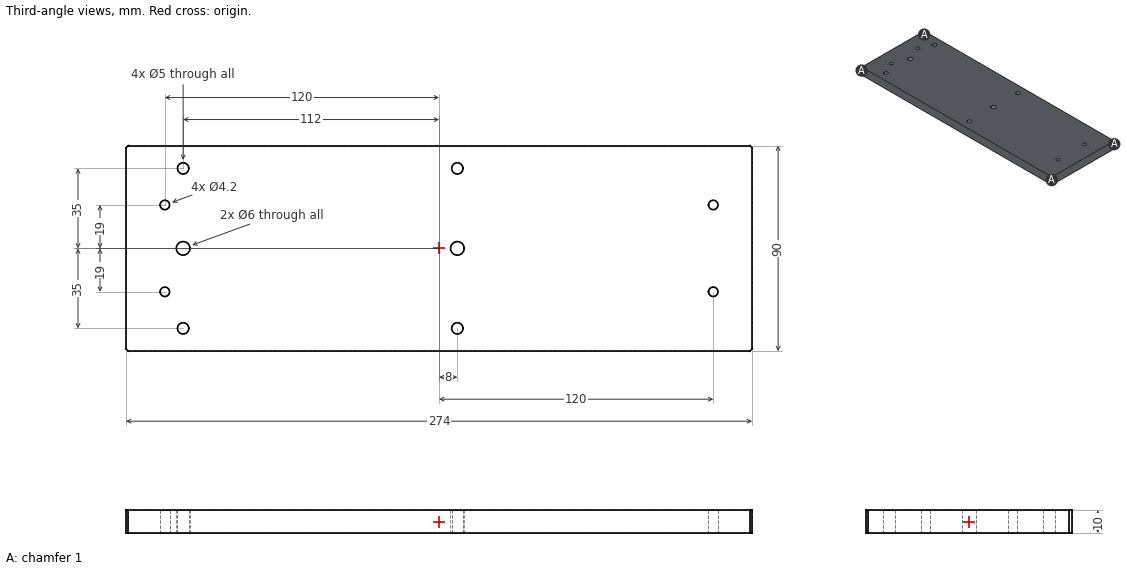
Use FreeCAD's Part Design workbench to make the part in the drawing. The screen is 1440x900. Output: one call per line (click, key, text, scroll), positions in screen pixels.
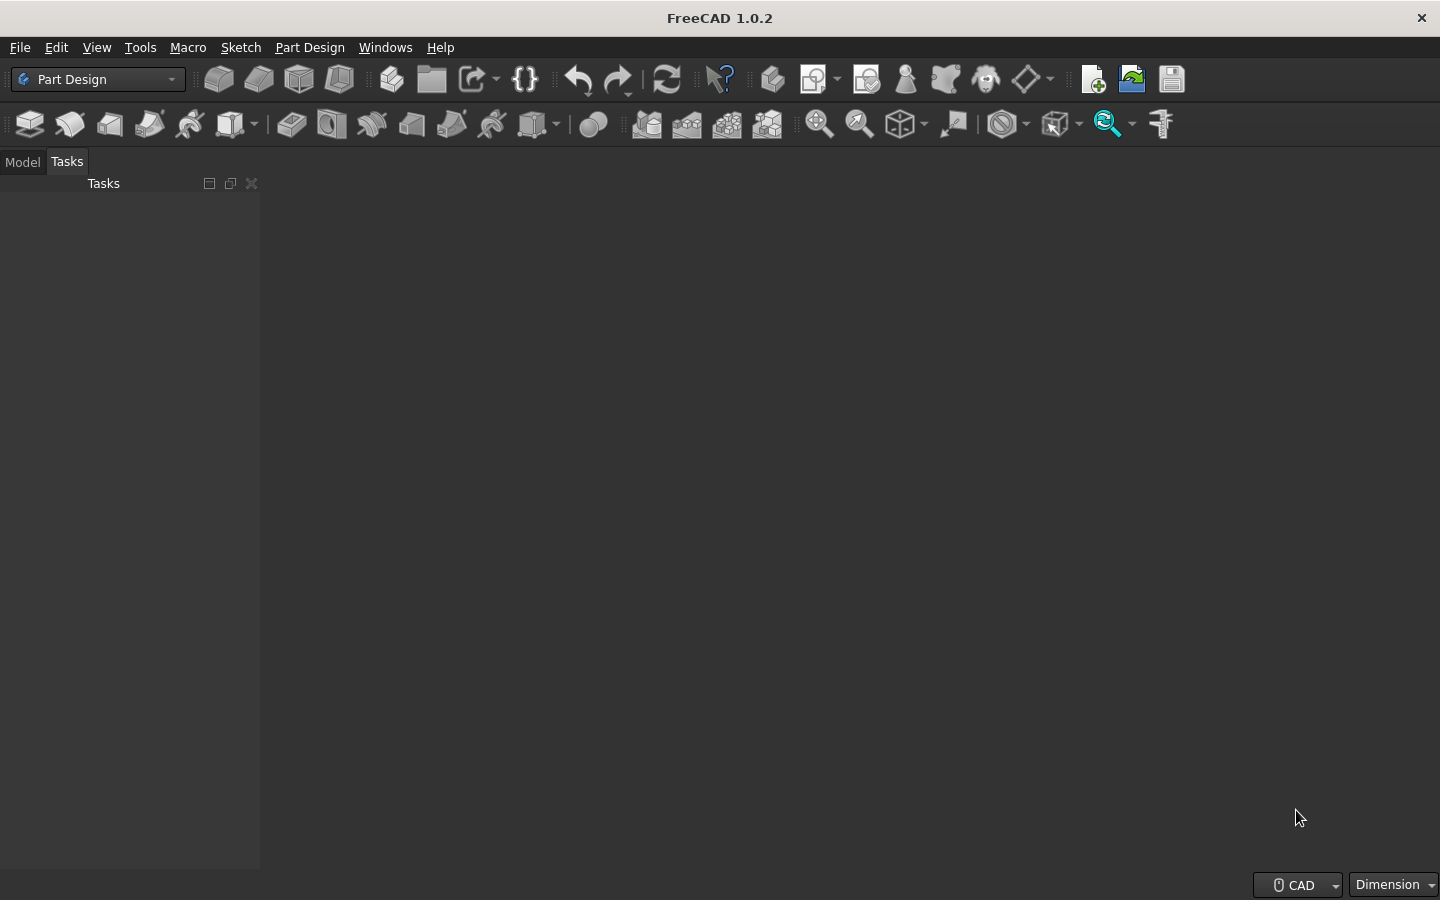
key(ctrl+n)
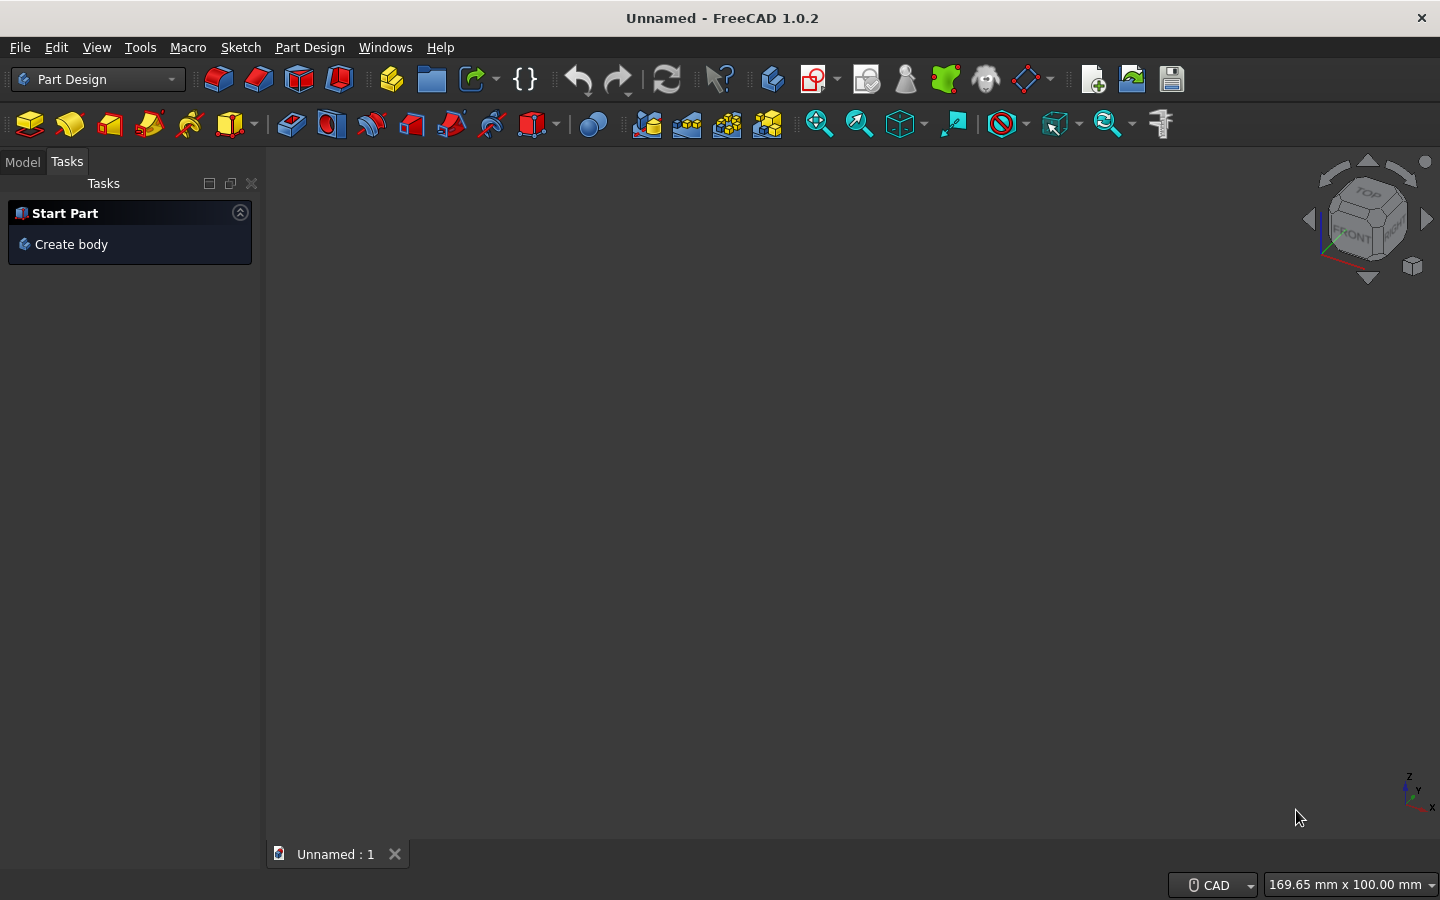
click(814, 80)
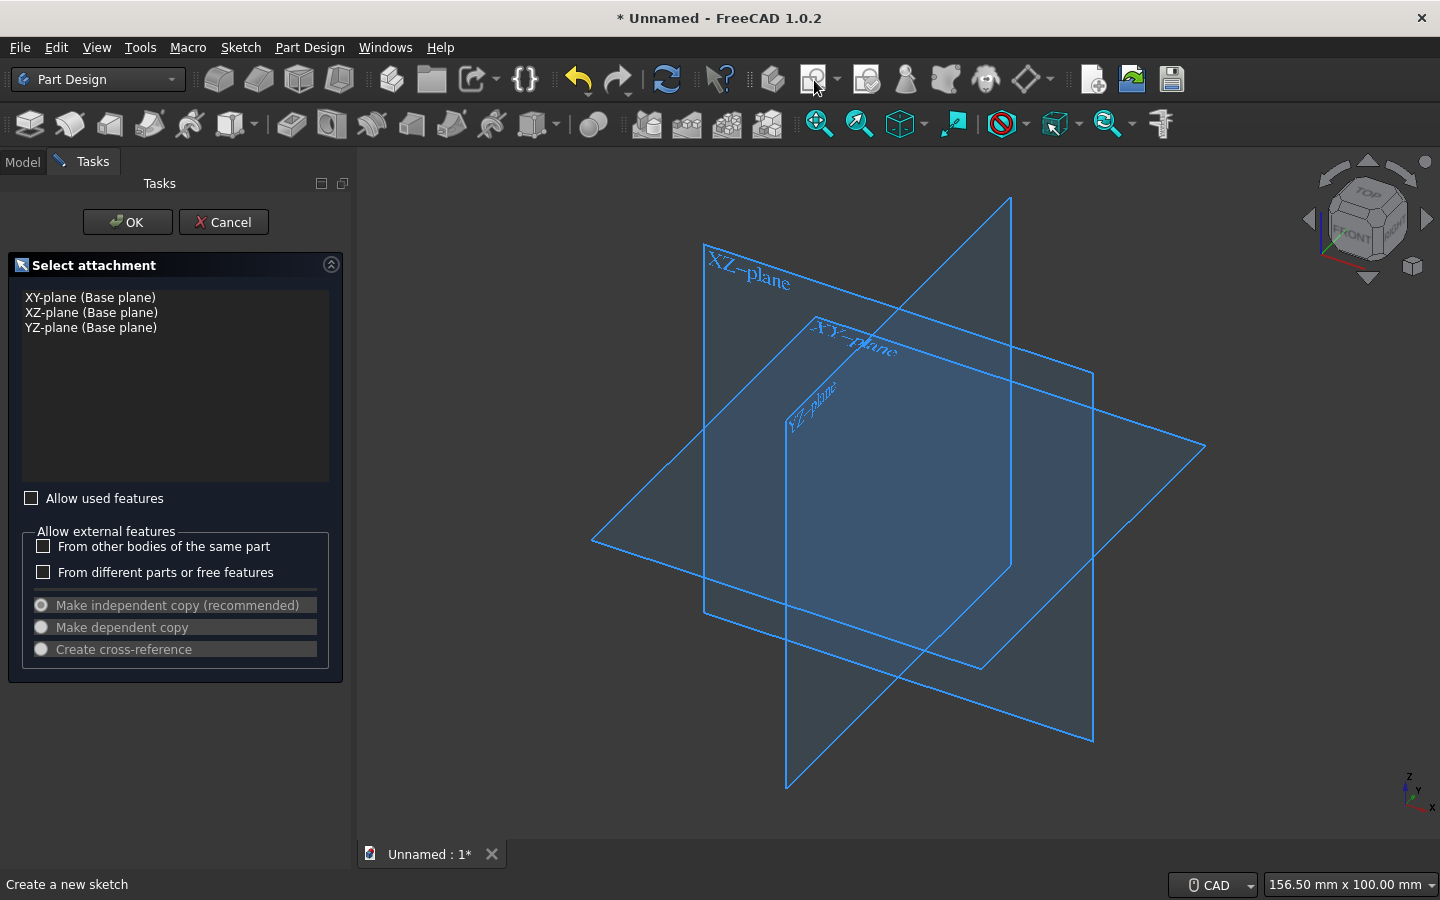
click(82, 298)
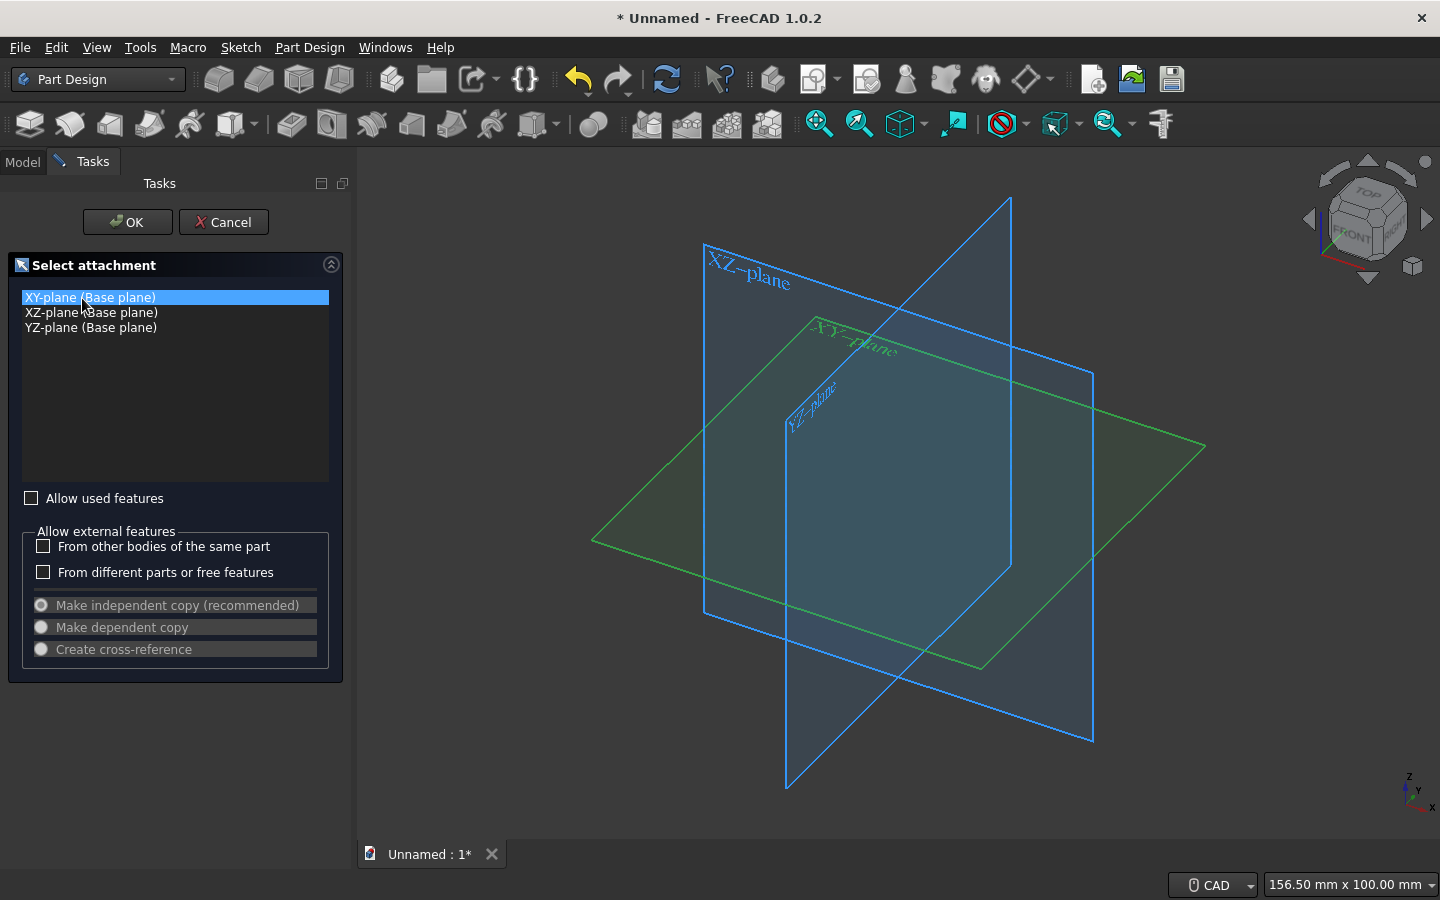
click(128, 222)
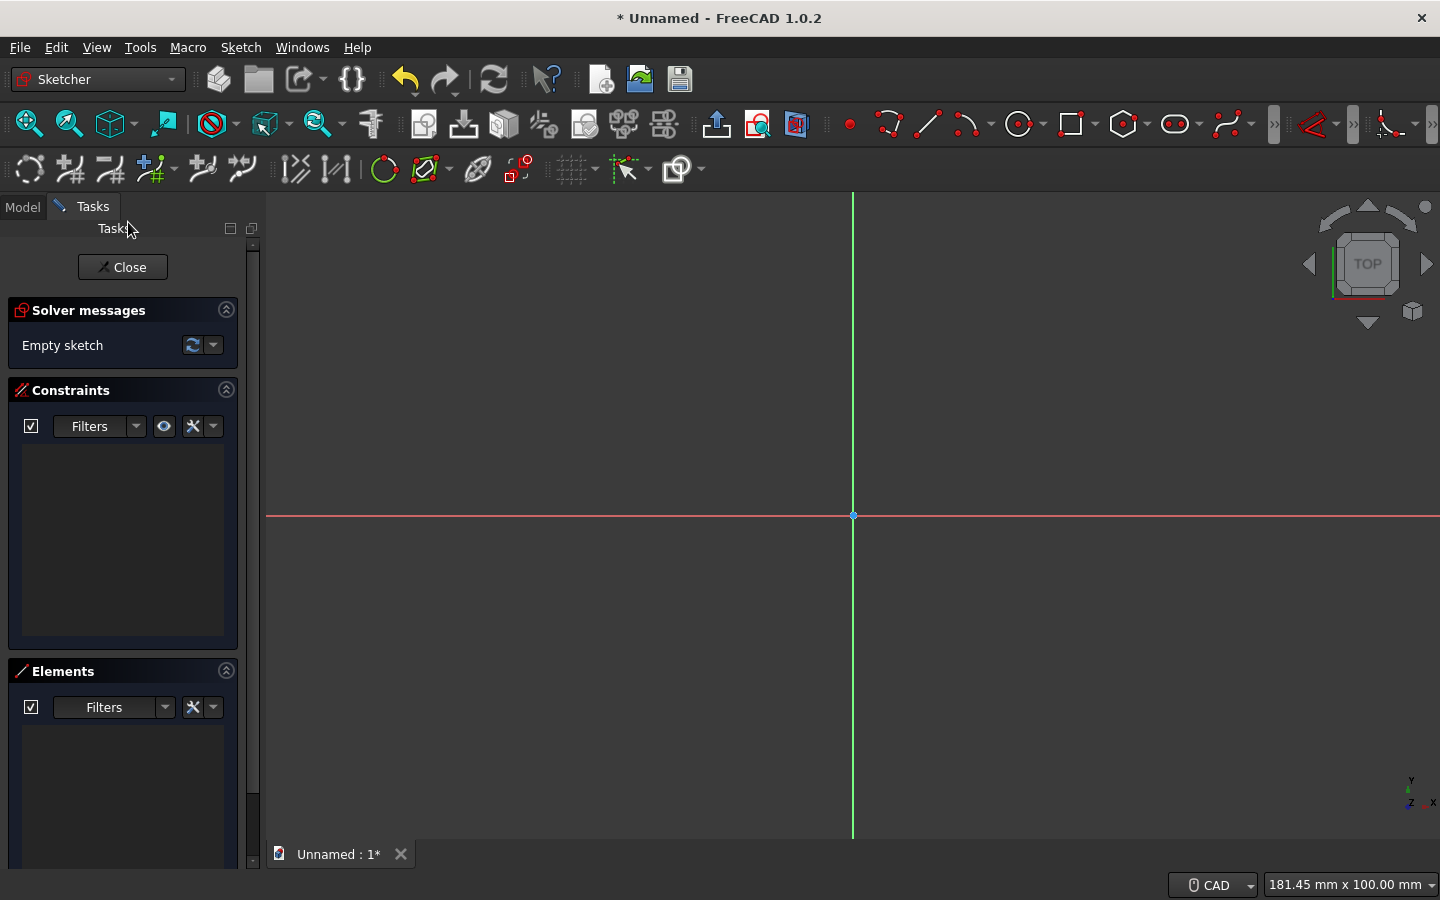
scroll(745, 515, down, 5)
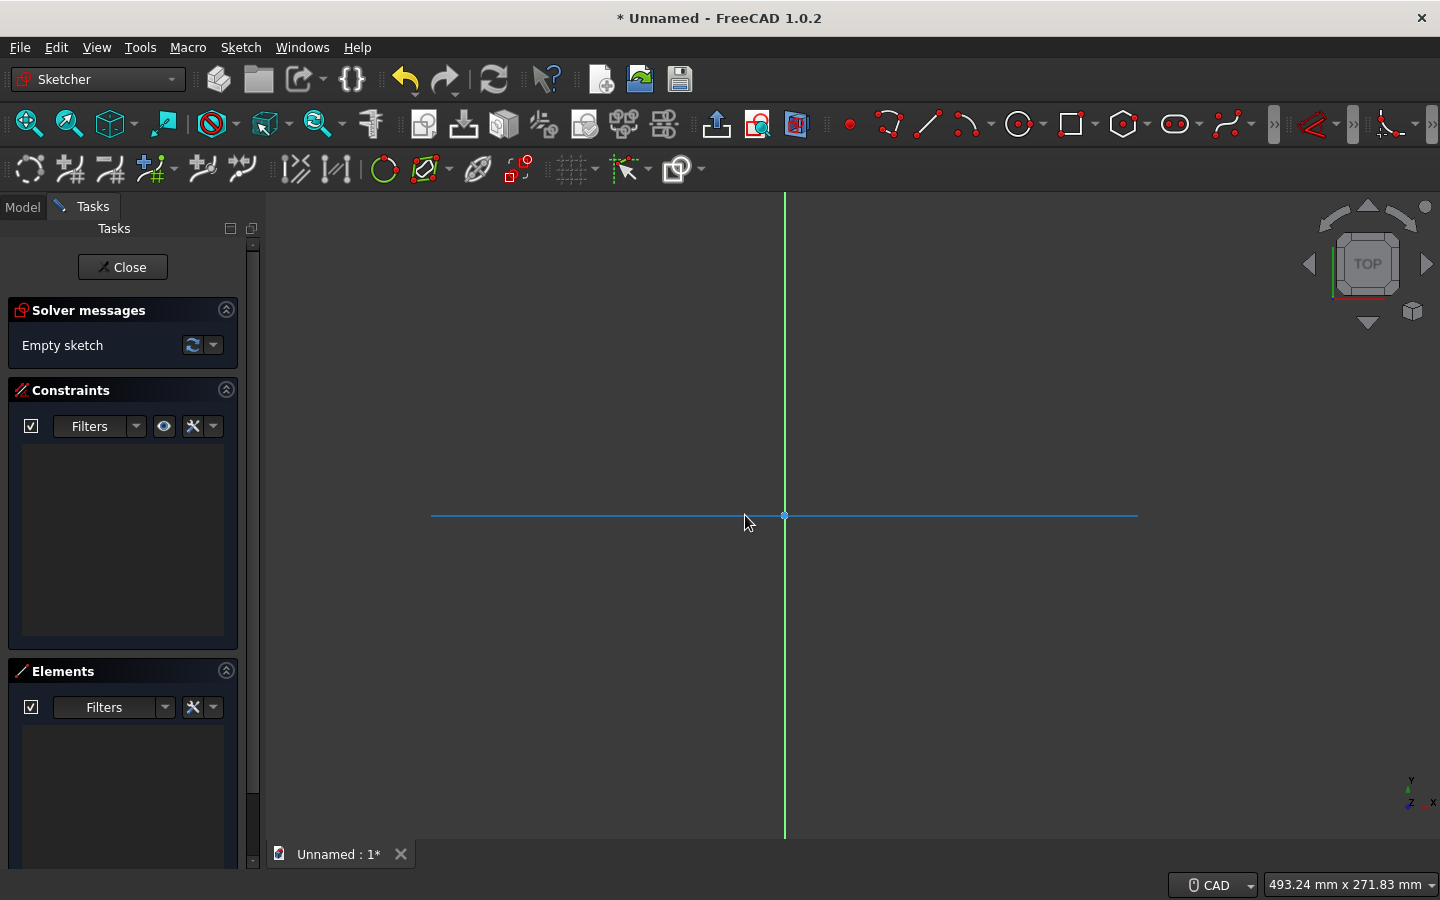
key(g)
key(v)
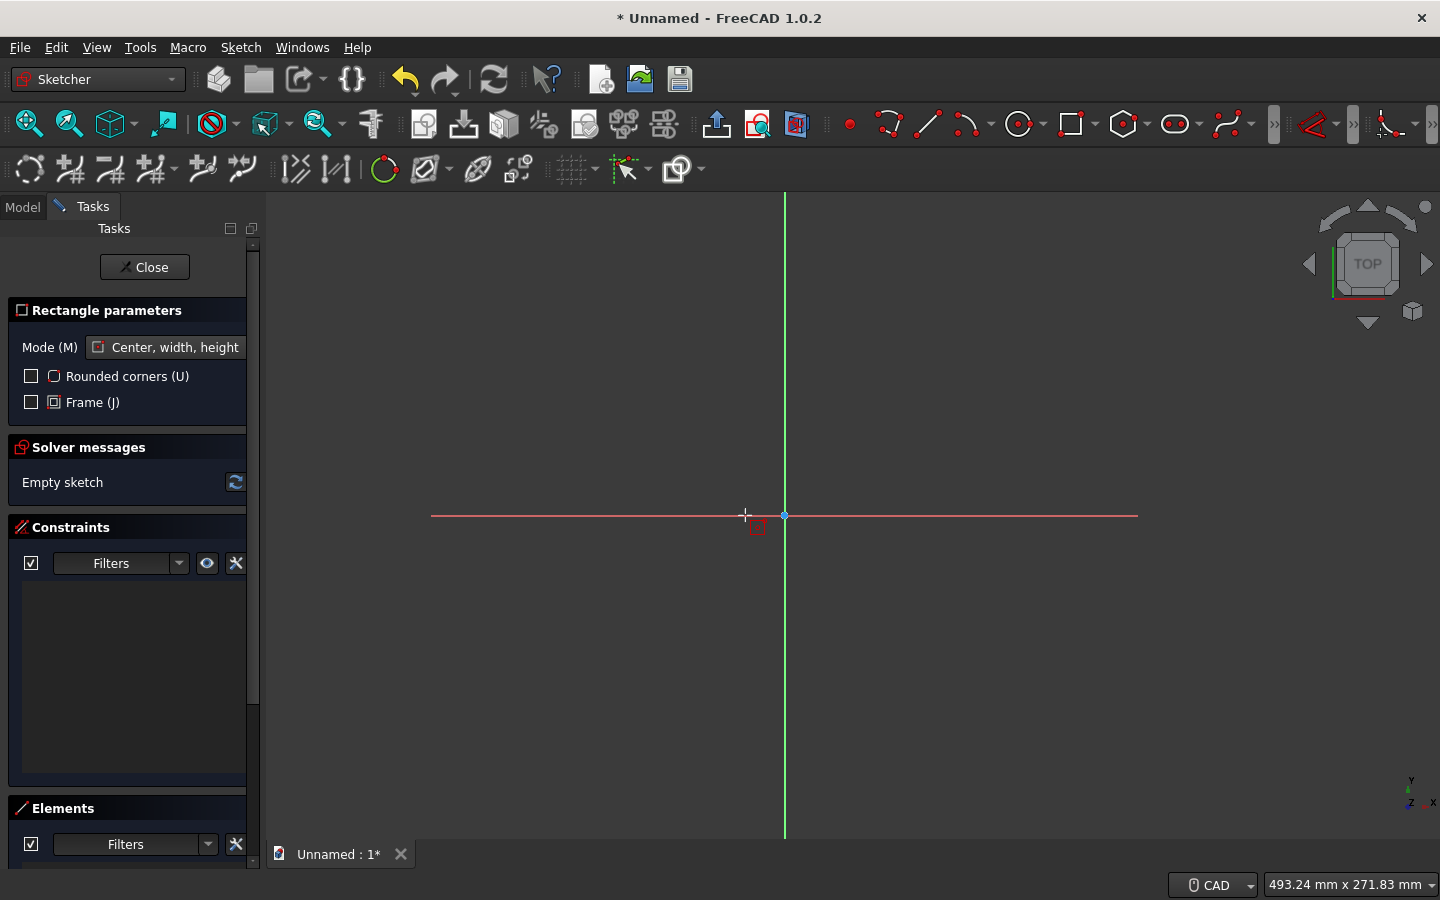
click(785, 516)
click(1111, 408)
key(Escape)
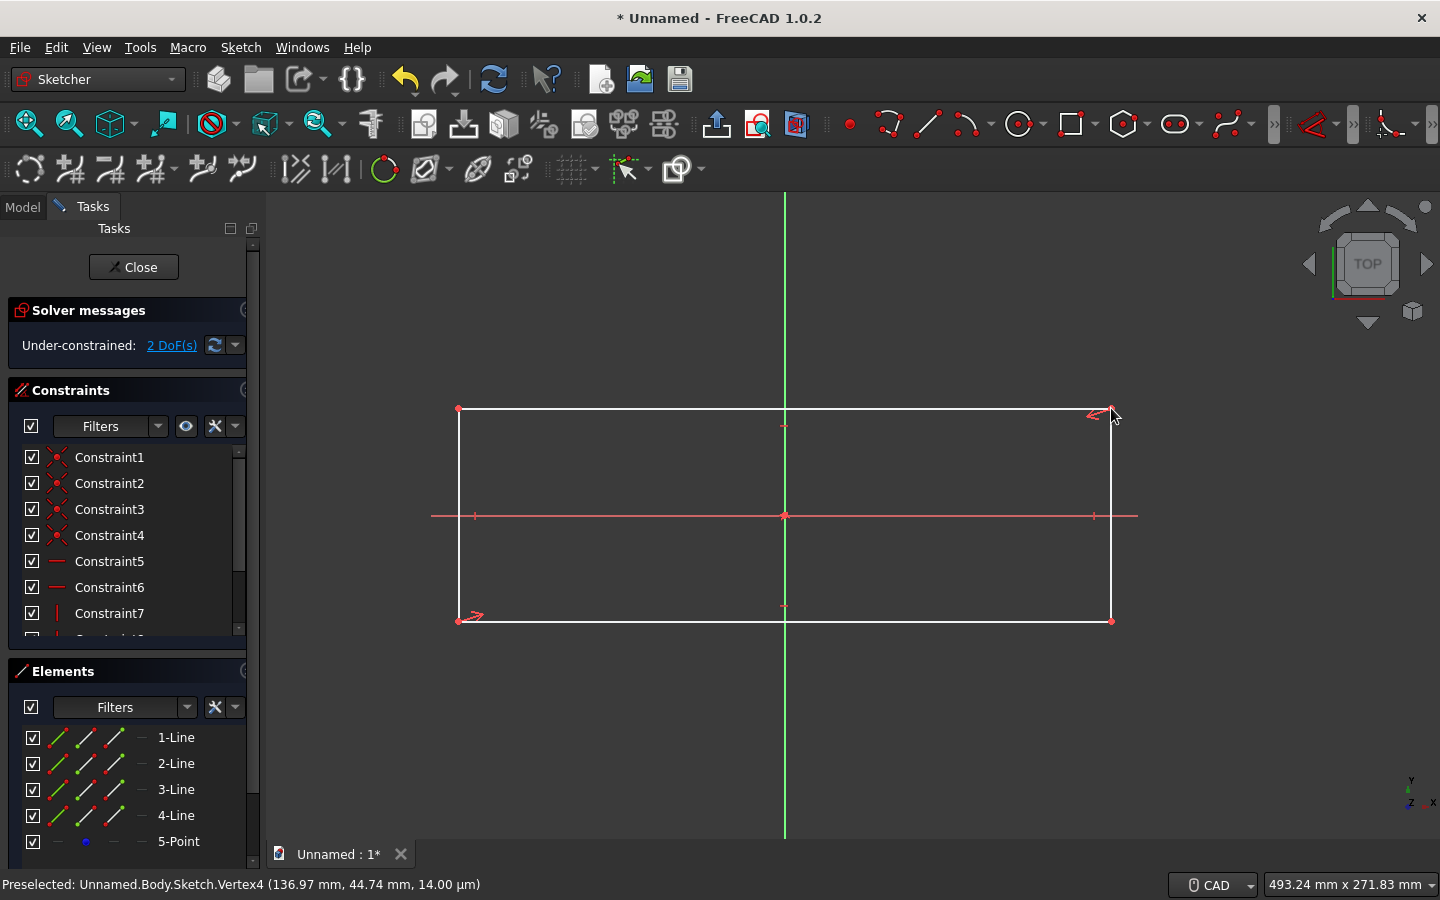
click(1111, 558)